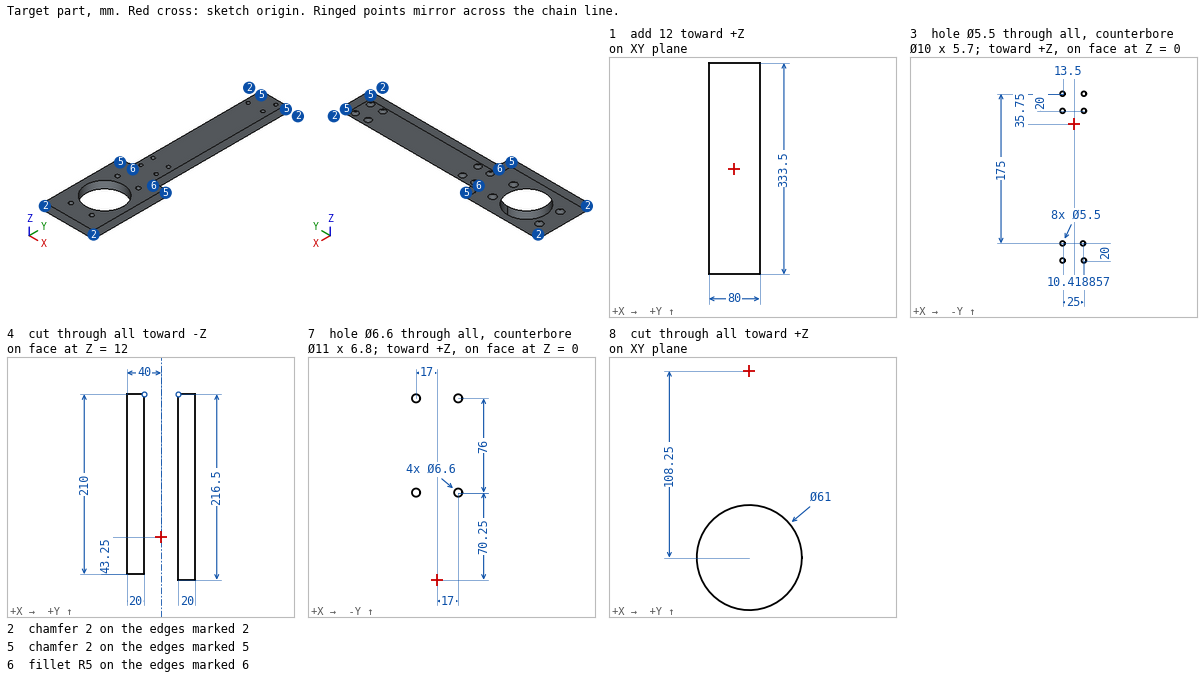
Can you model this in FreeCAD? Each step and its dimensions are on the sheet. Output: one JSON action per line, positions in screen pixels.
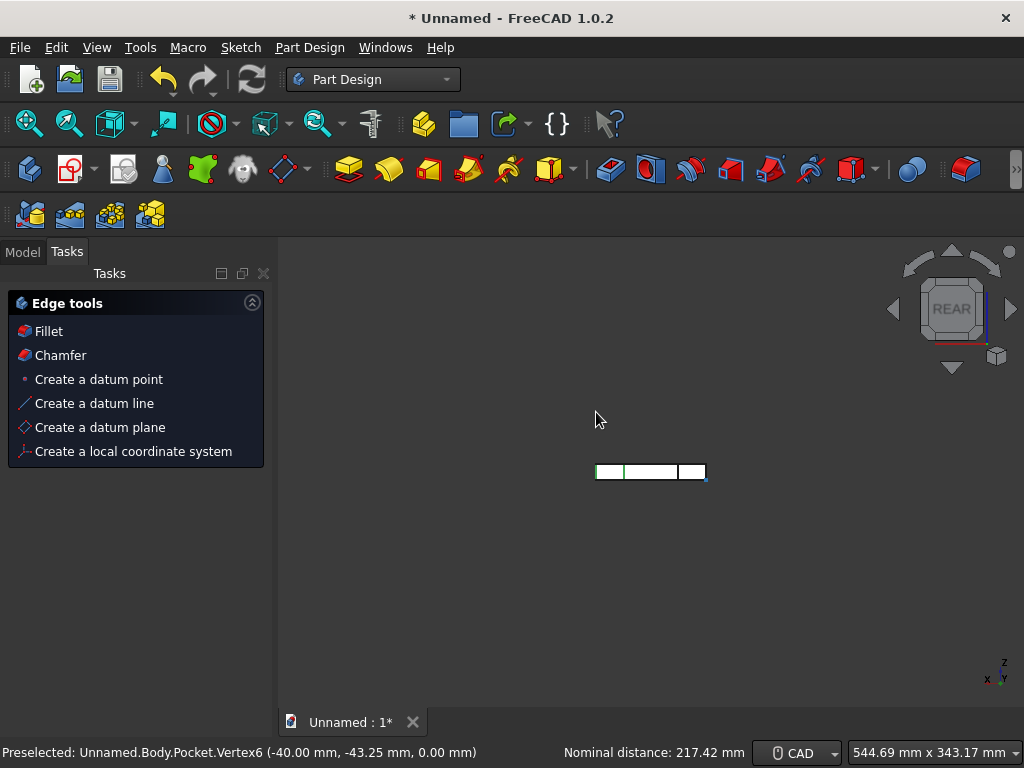
{"action": "left_click", "coordinate": [706, 471], "text": "ctrl"}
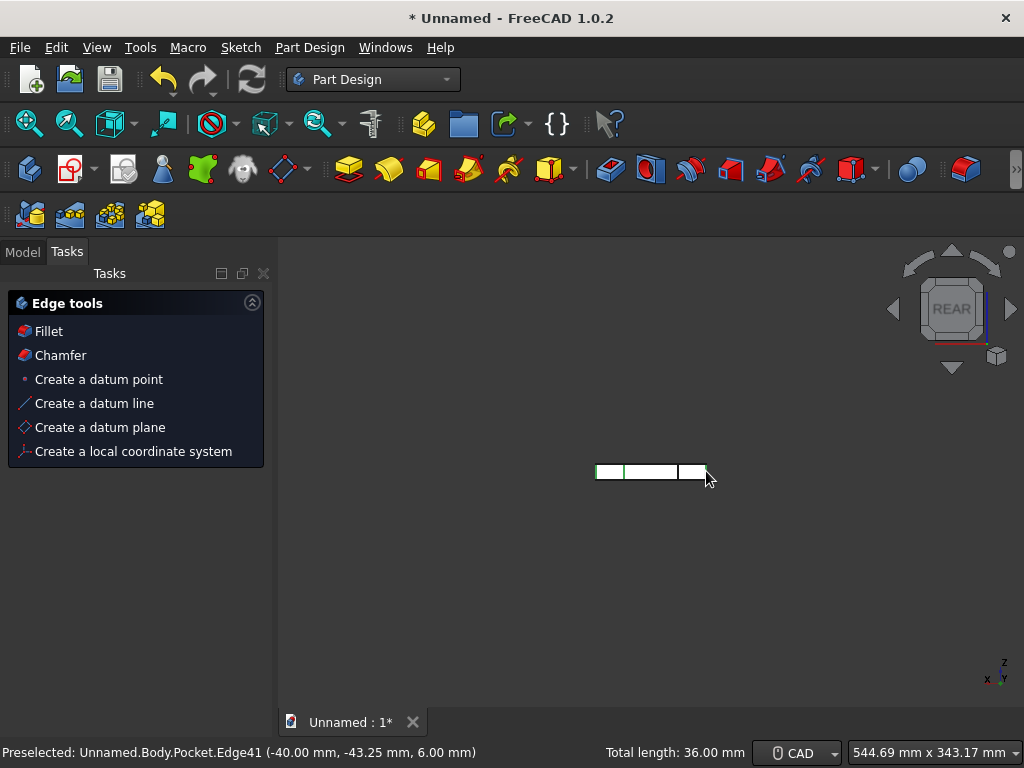
{"action": "left_click", "coordinate": [678, 471], "text": "ctrl"}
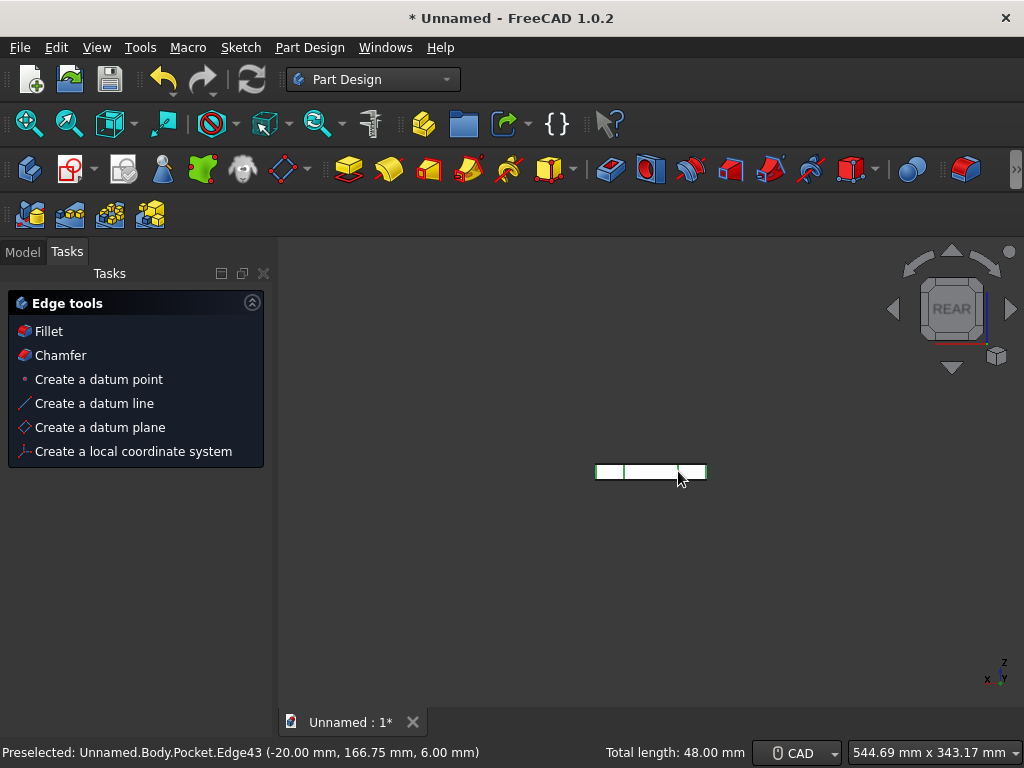
{"action": "left_click", "coordinate": [136, 355]}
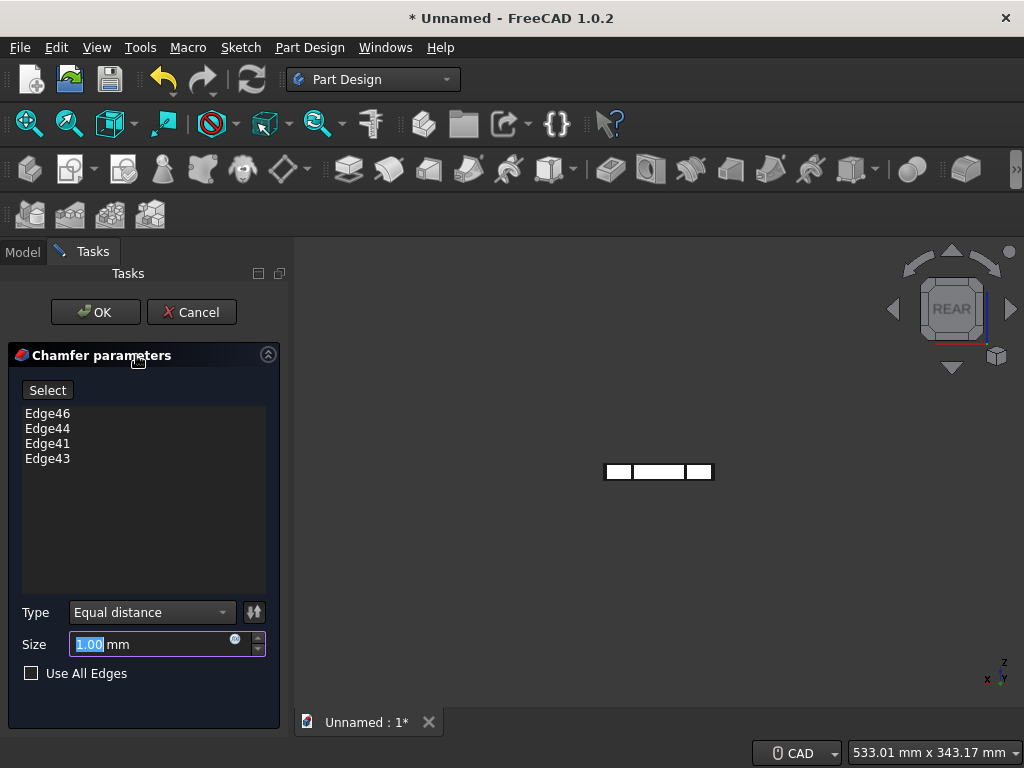
{"action": "type", "text": "2"}
{"action": "key", "text": "Tab"}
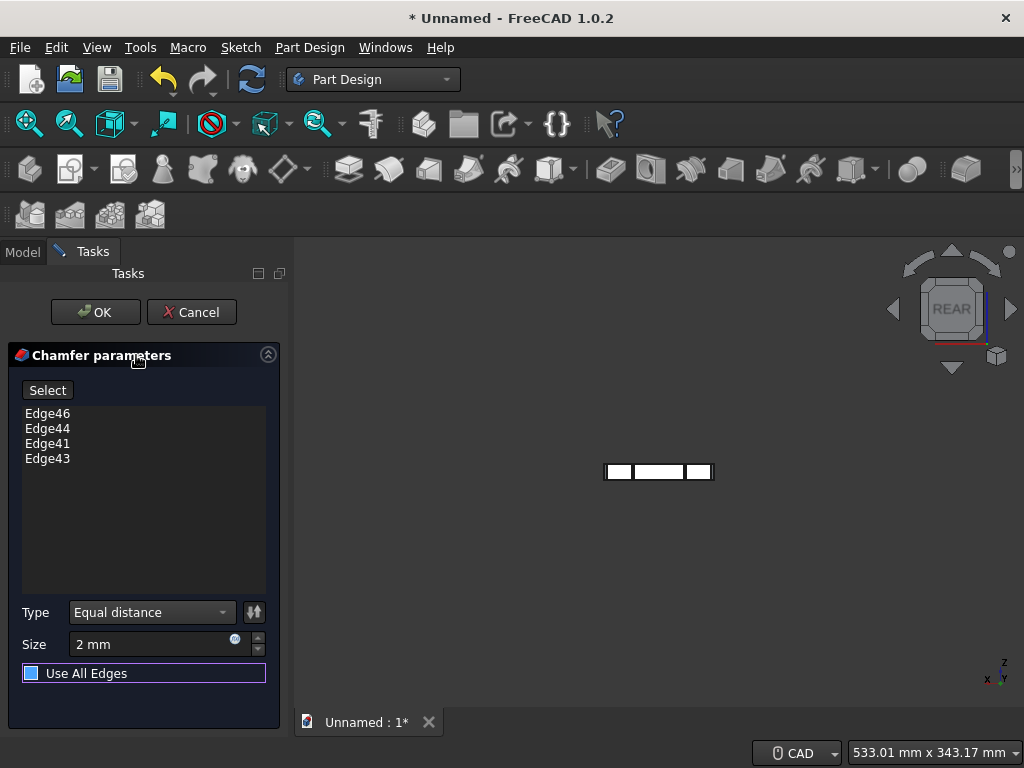
{"action": "left_click", "coordinate": [96, 312]}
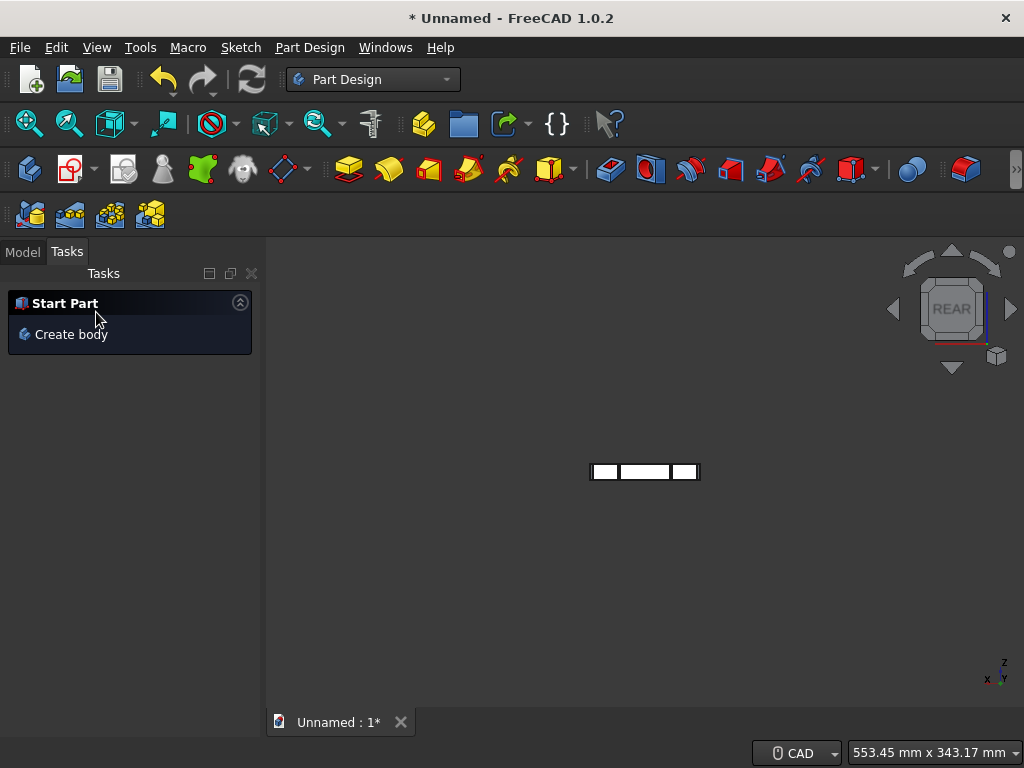
{"action": "key", "text": "v f"}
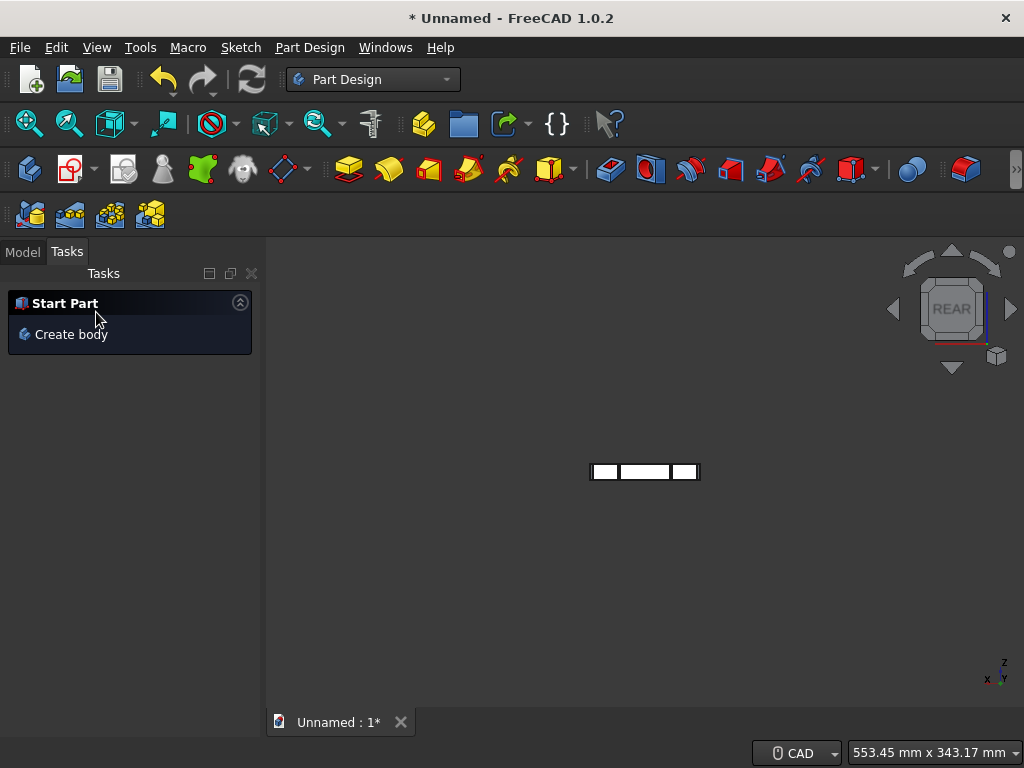
{"action": "scroll", "coordinate": [672, 471], "scroll_direction": "up", "scroll_amount": 5}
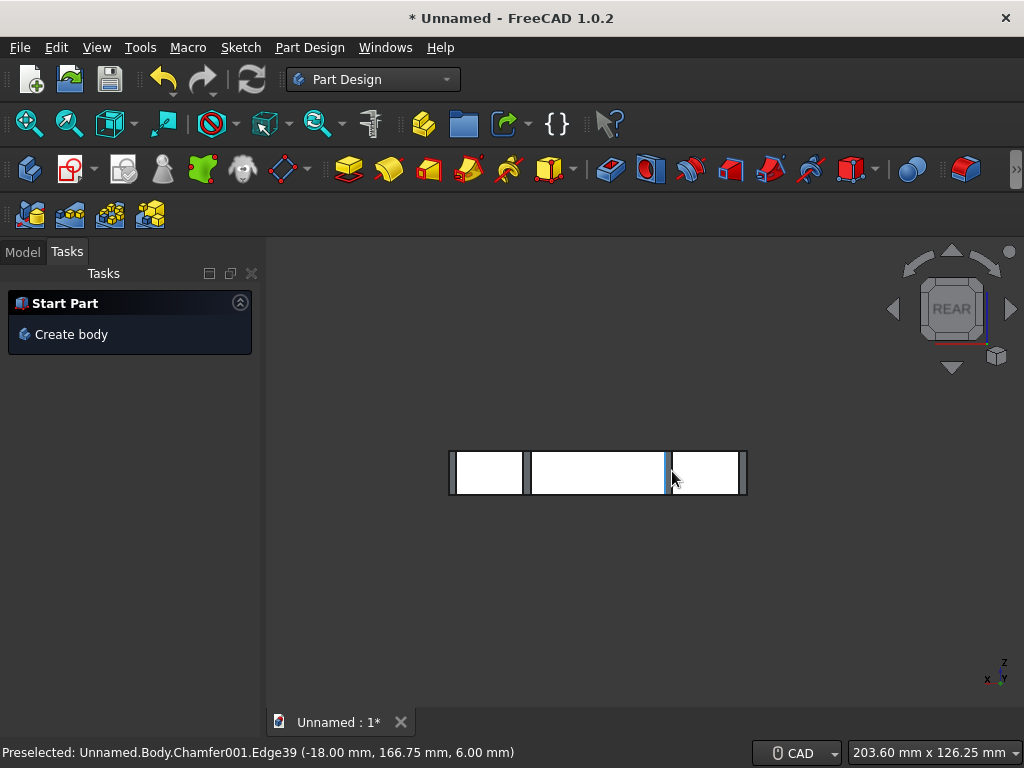
{"action": "left_click", "coordinate": [30, 124]}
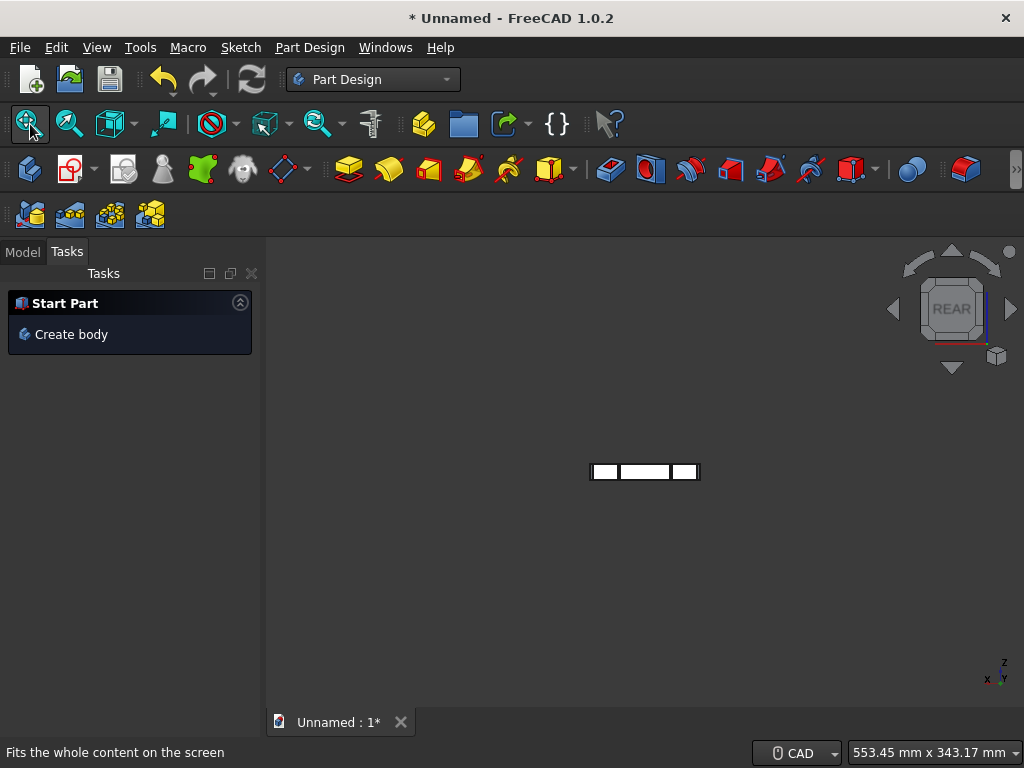
{"action": "key", "text": "0"}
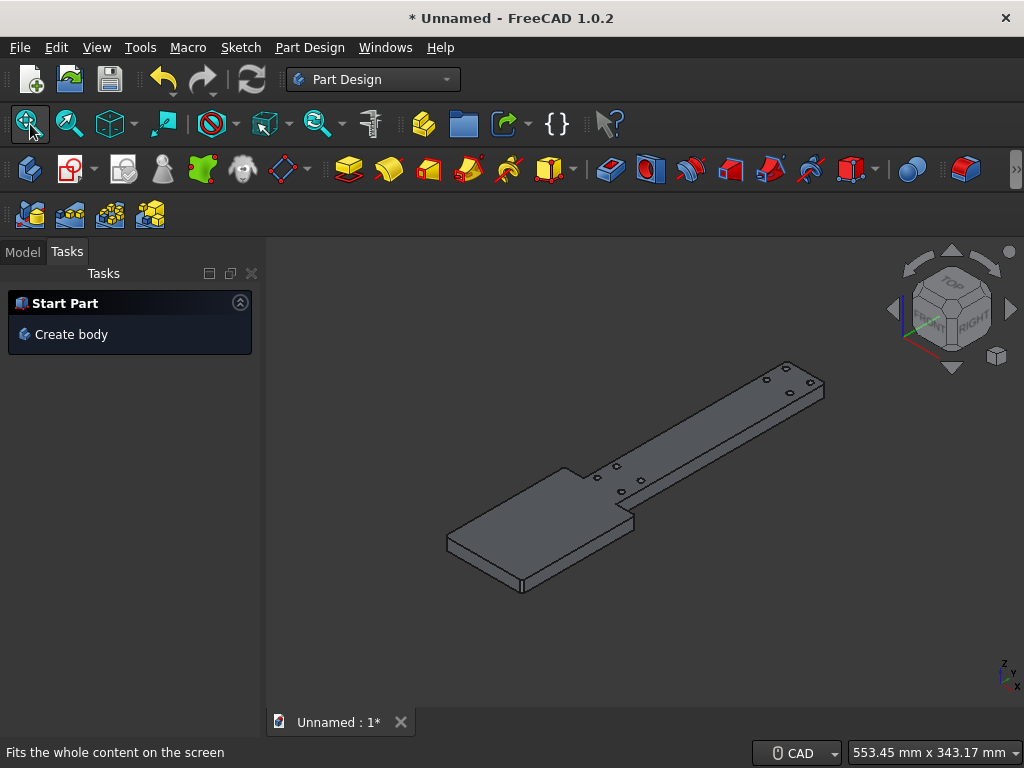
{"action": "scroll", "coordinate": [584, 484], "scroll_direction": "up", "scroll_amount": 5}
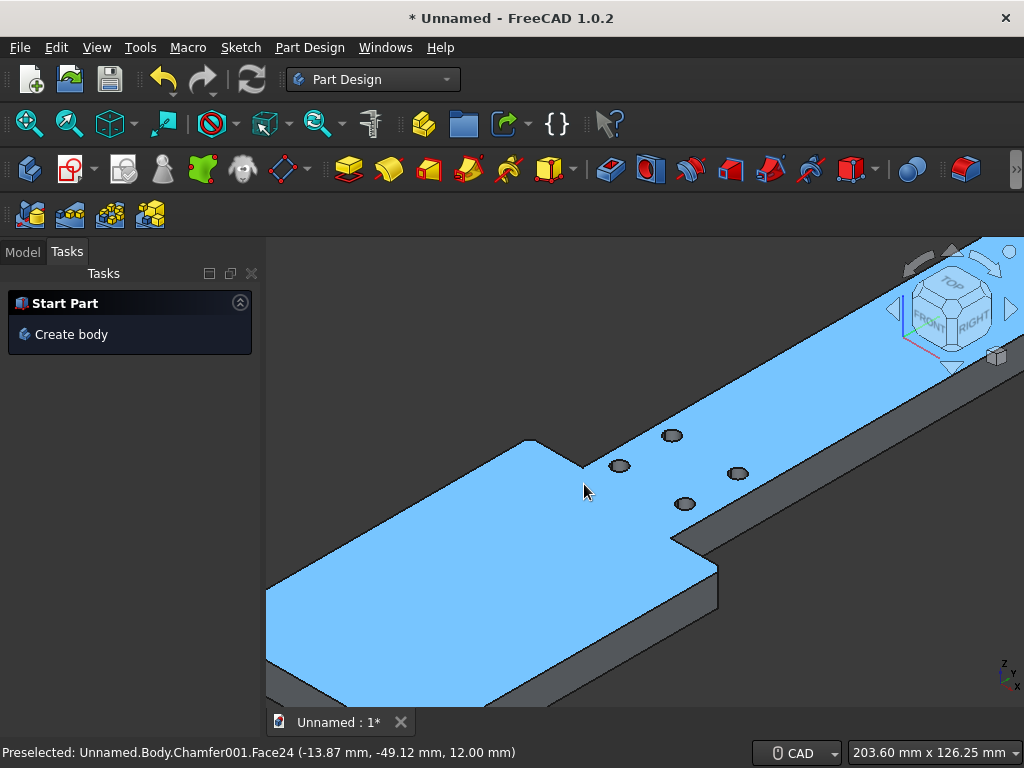
{"action": "key", "text": "v f"}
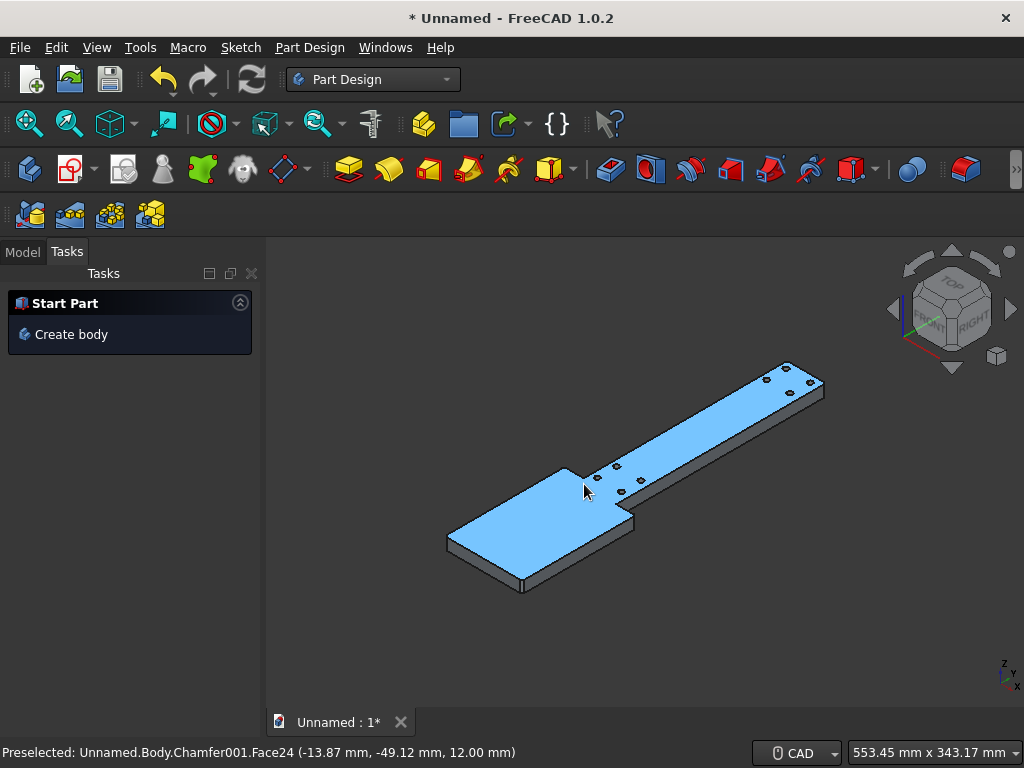
{"action": "key", "text": "2"}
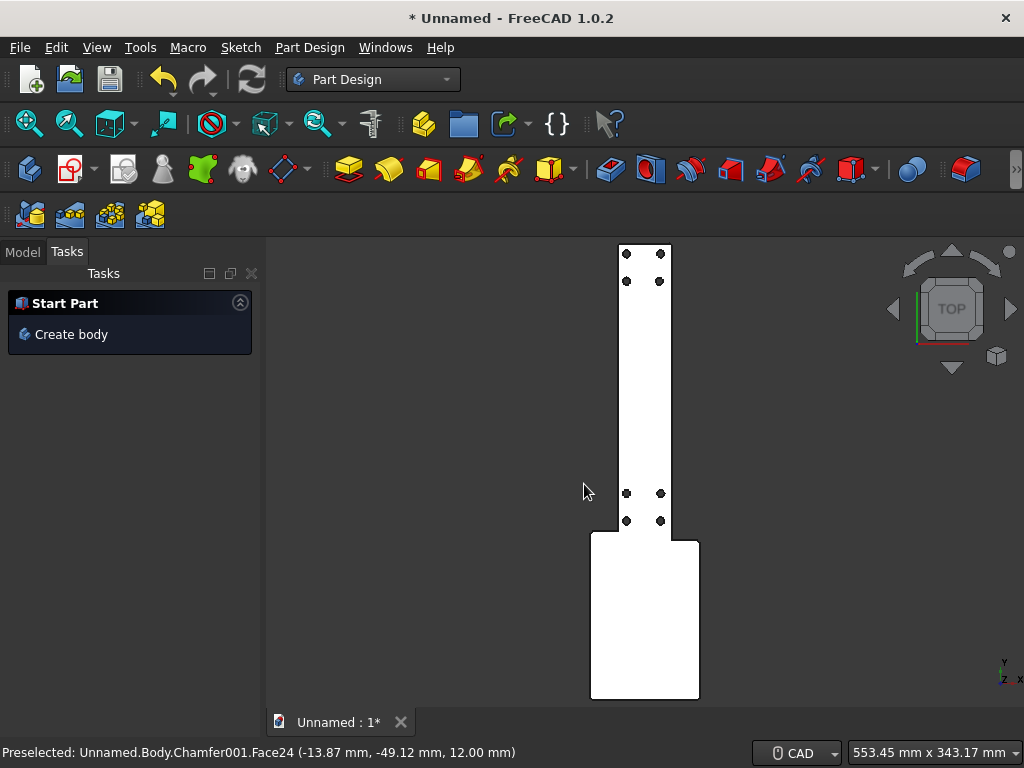
{"action": "scroll", "coordinate": [618, 530], "scroll_direction": "up", "scroll_amount": 5}